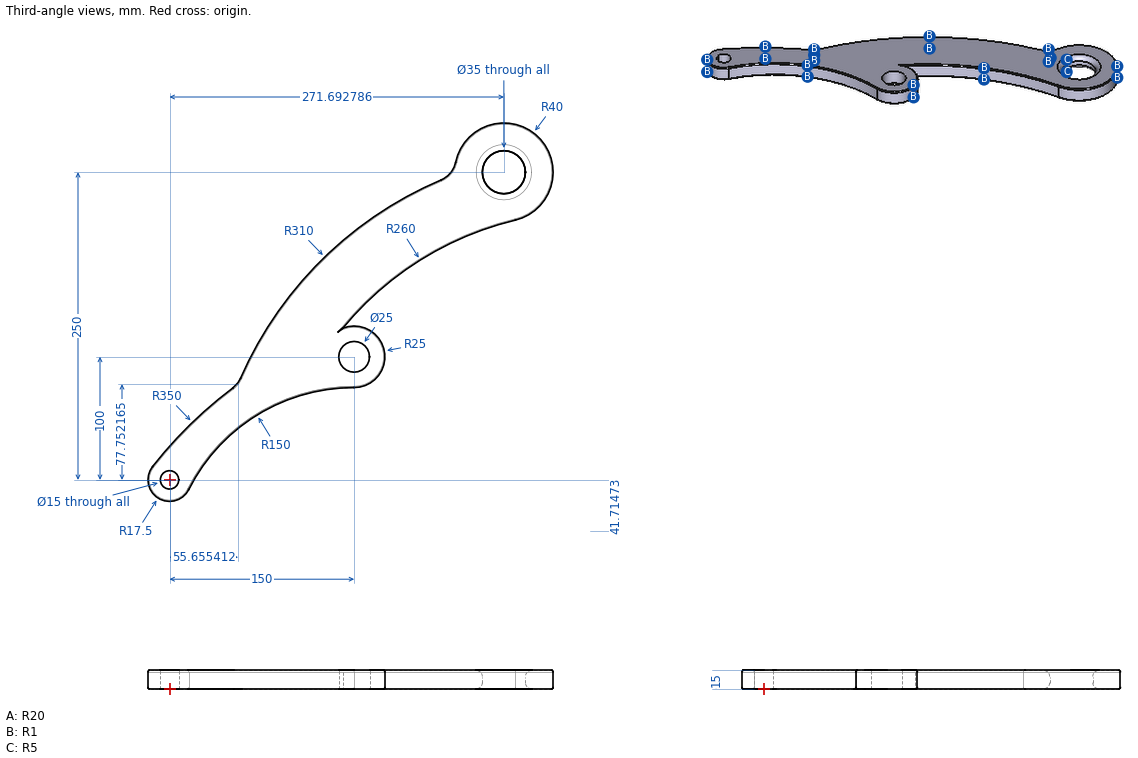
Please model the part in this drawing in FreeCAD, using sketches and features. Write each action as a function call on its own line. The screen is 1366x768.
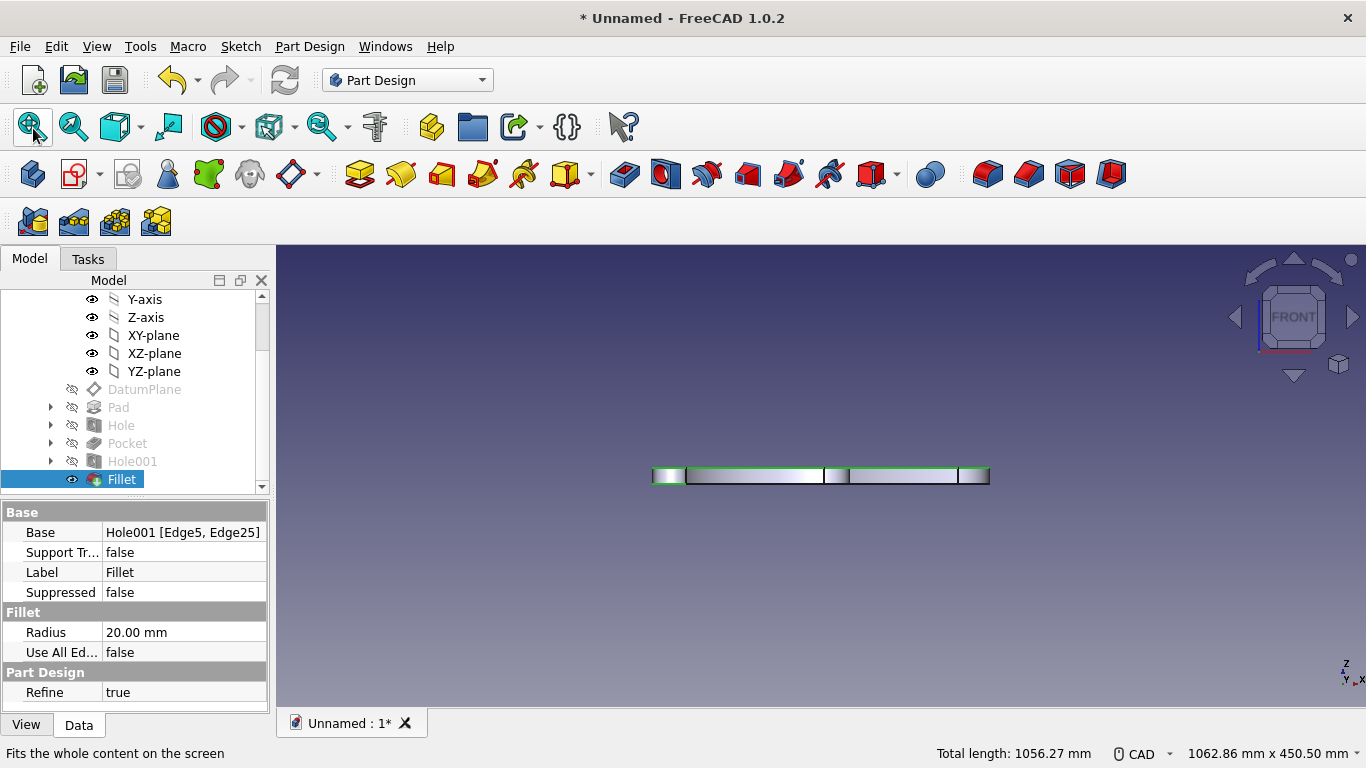
click(743, 483, ctrl)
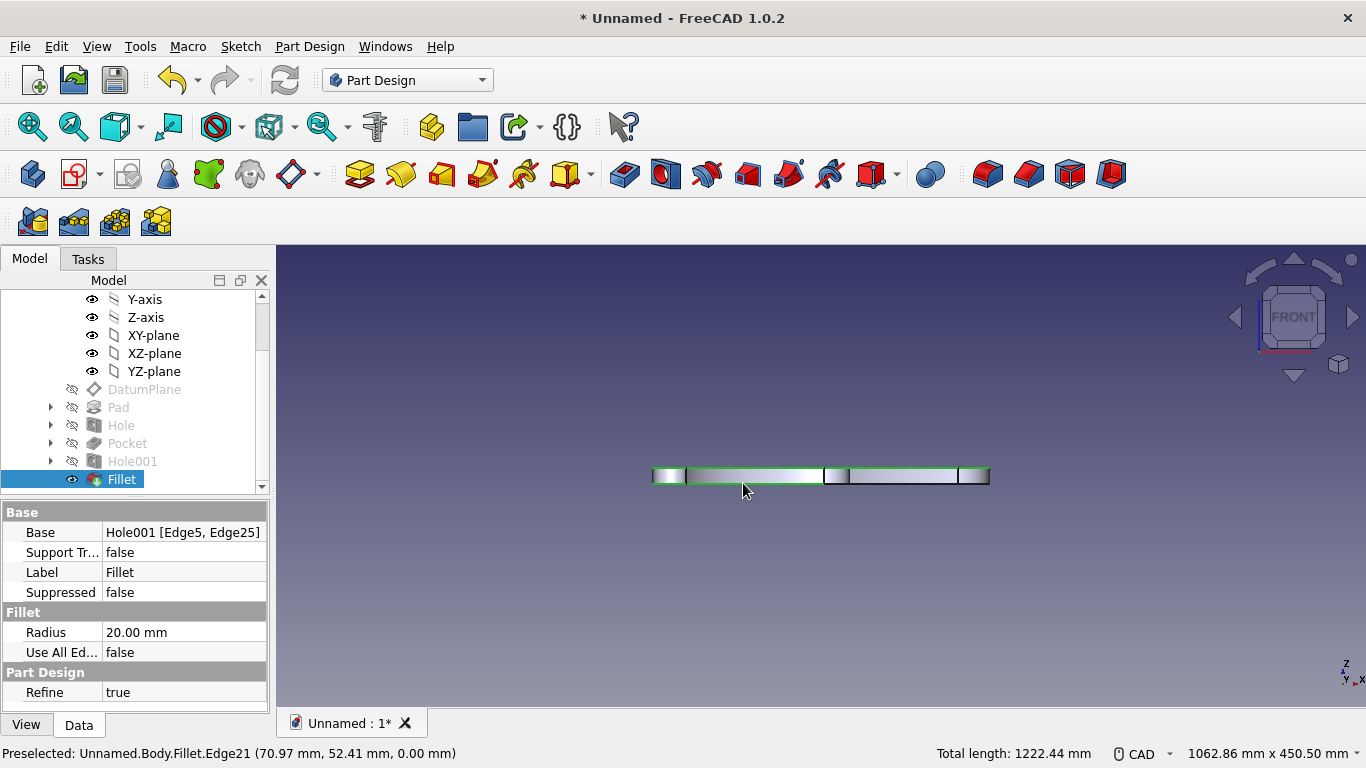
click(849, 483, ctrl)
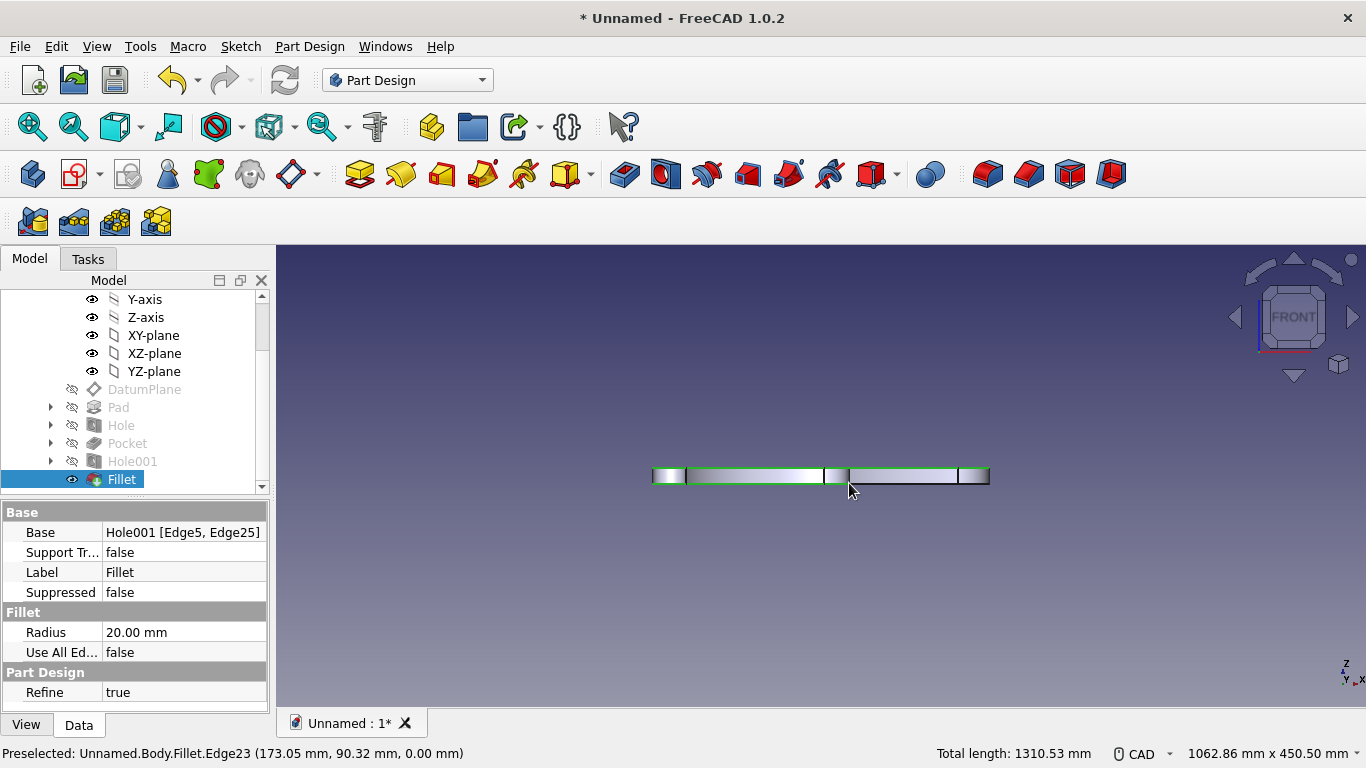
click(879, 483, ctrl)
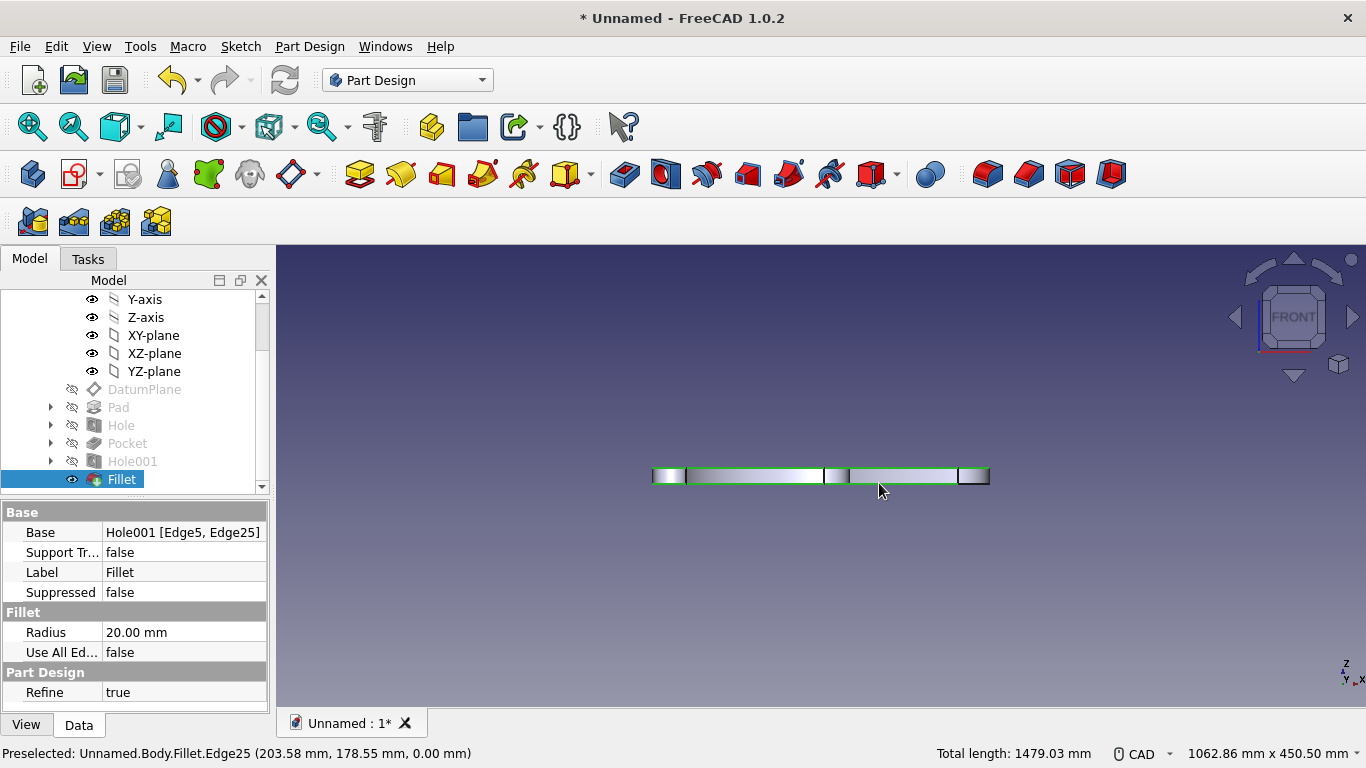
click(977, 483, ctrl)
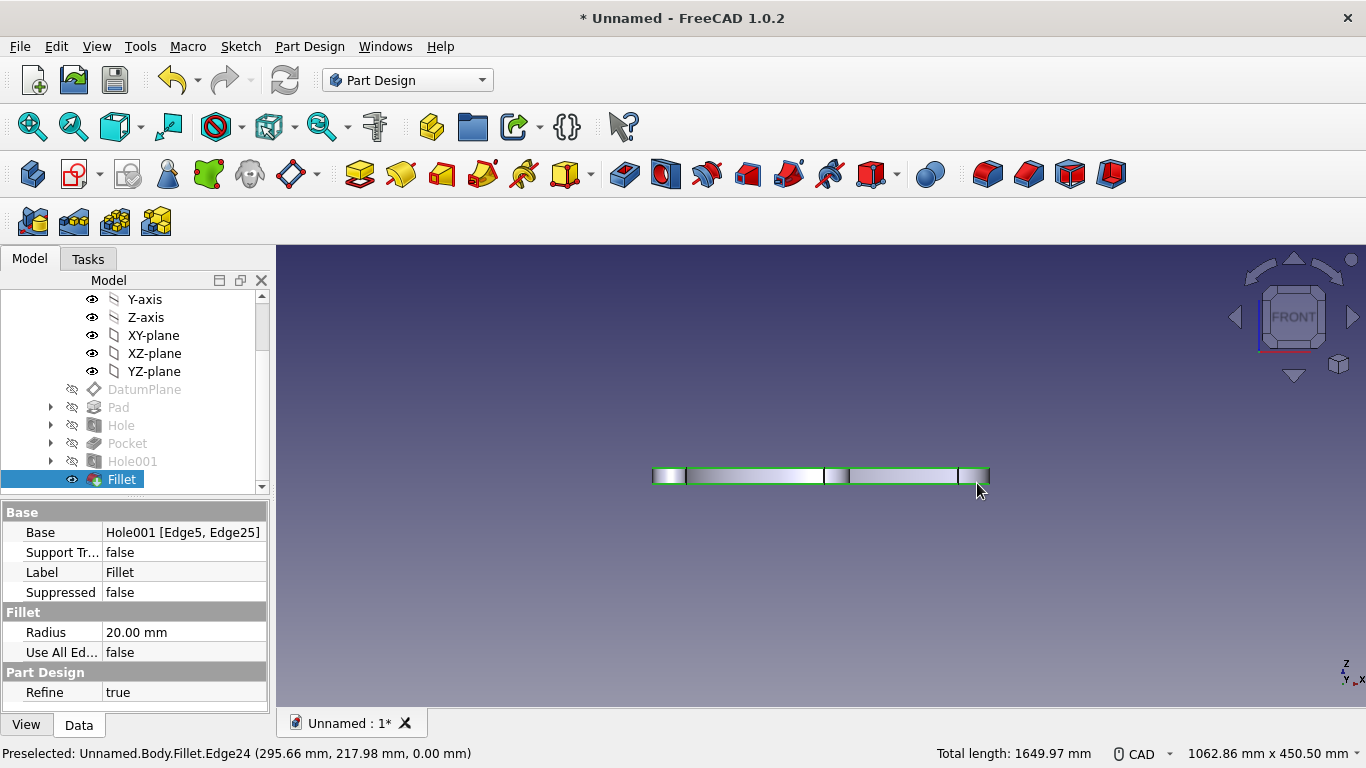
key(3)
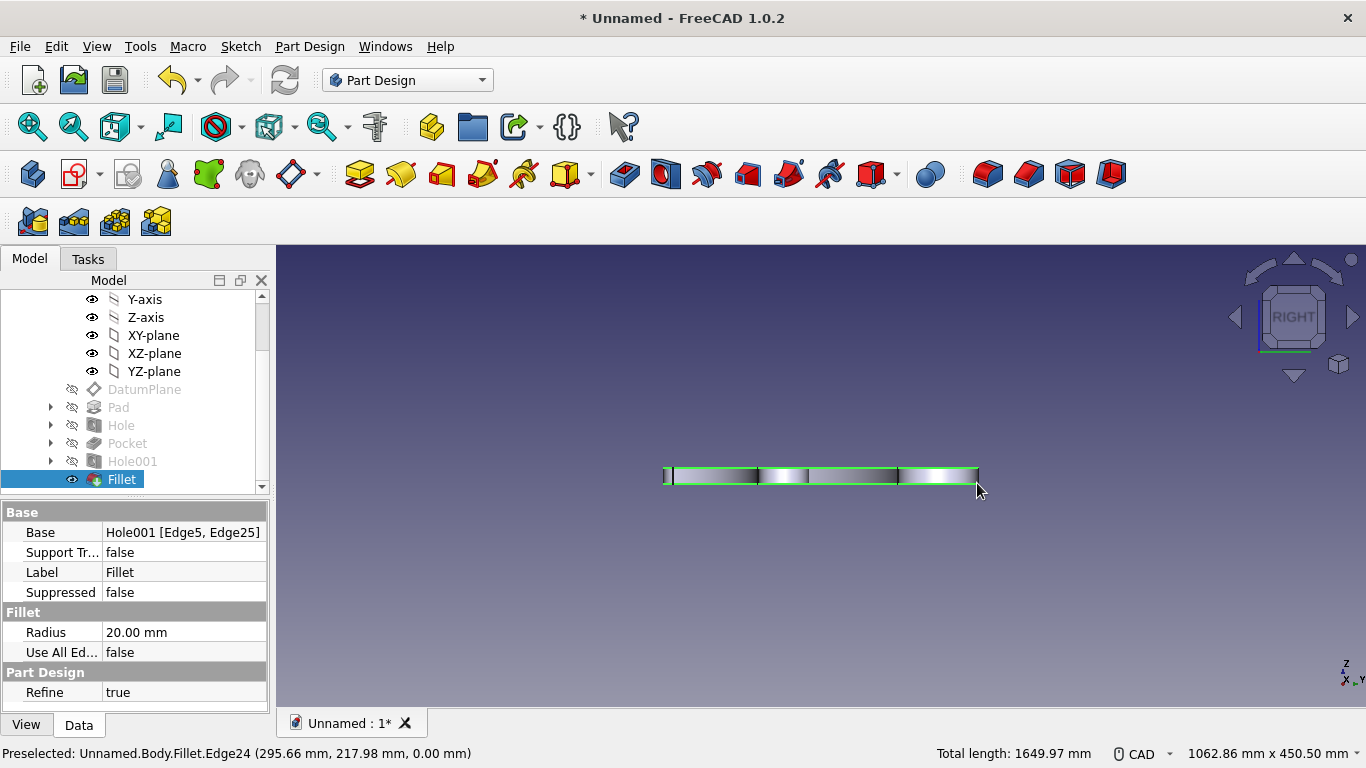
click(33, 128)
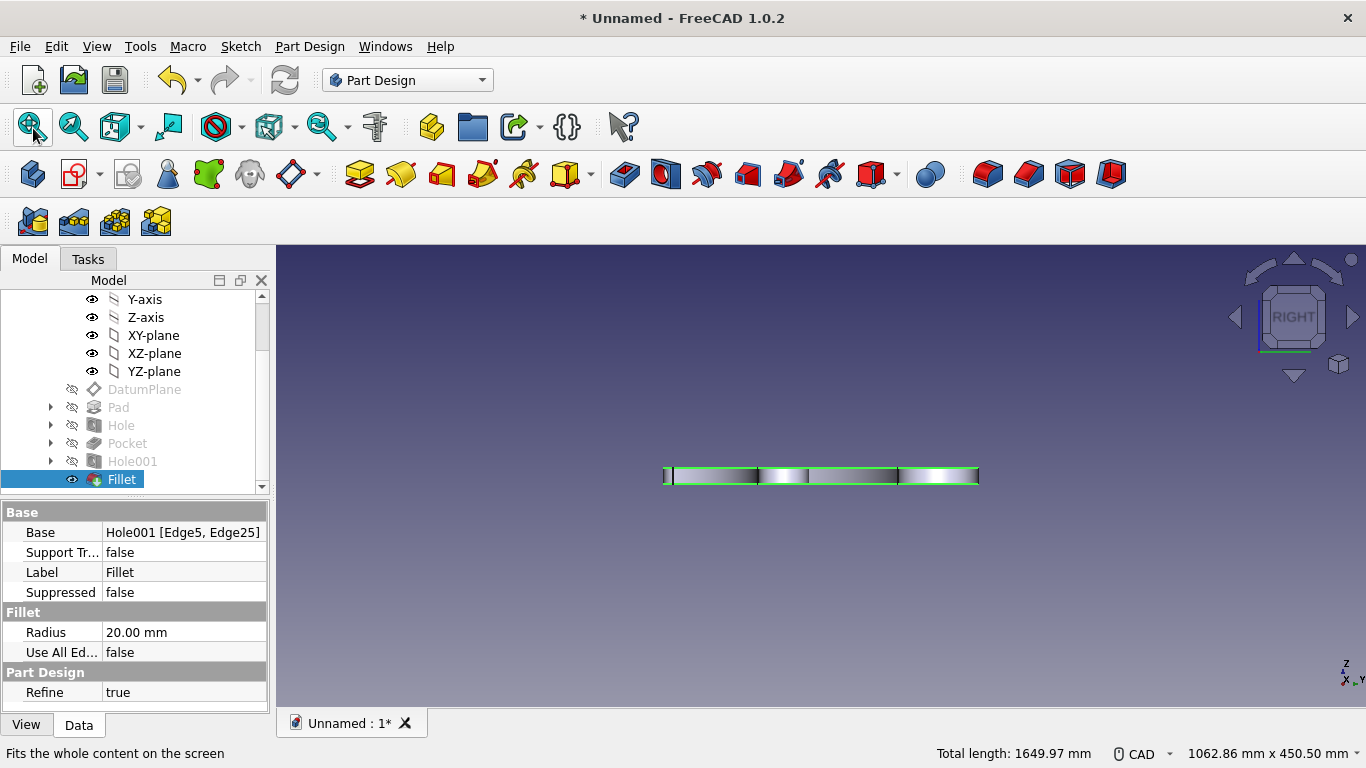
key(5)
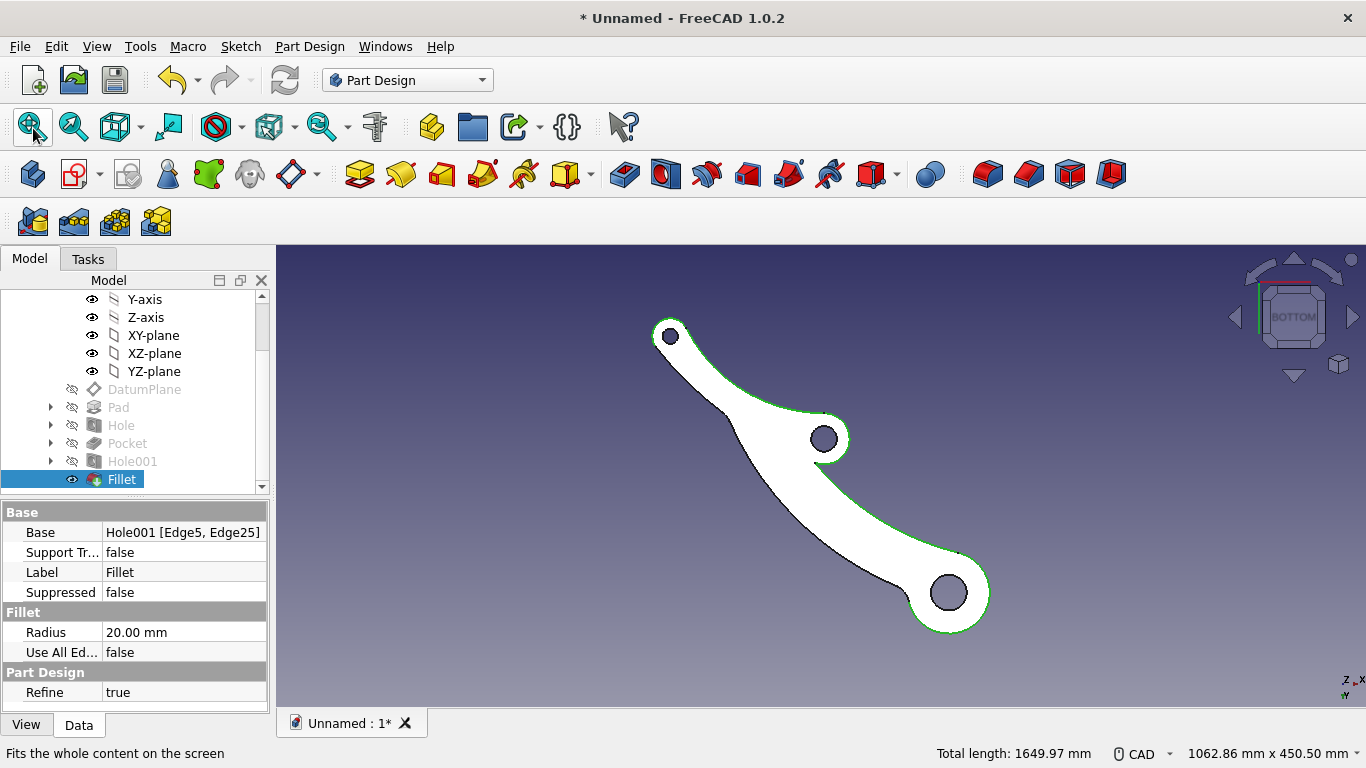
click(797, 519, ctrl)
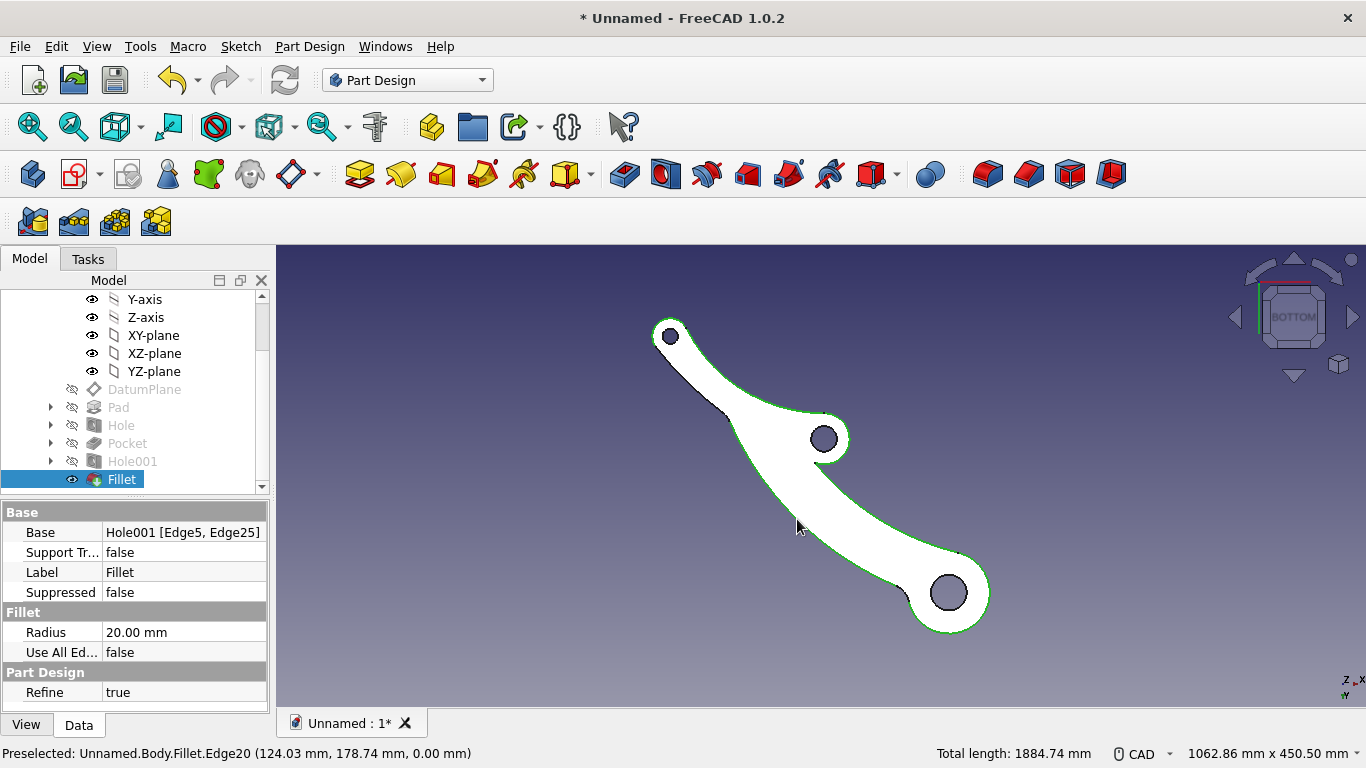
click(687, 381, ctrl)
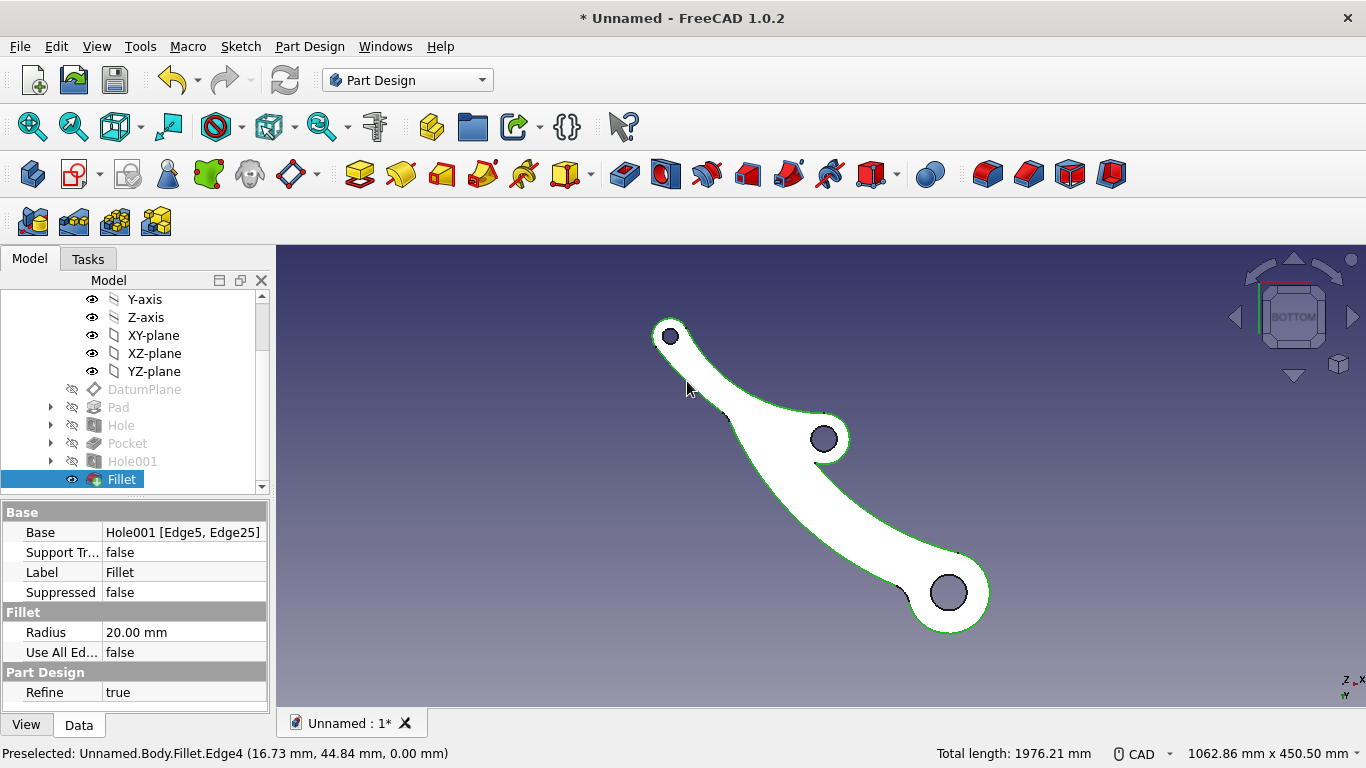
click(904, 591, ctrl)